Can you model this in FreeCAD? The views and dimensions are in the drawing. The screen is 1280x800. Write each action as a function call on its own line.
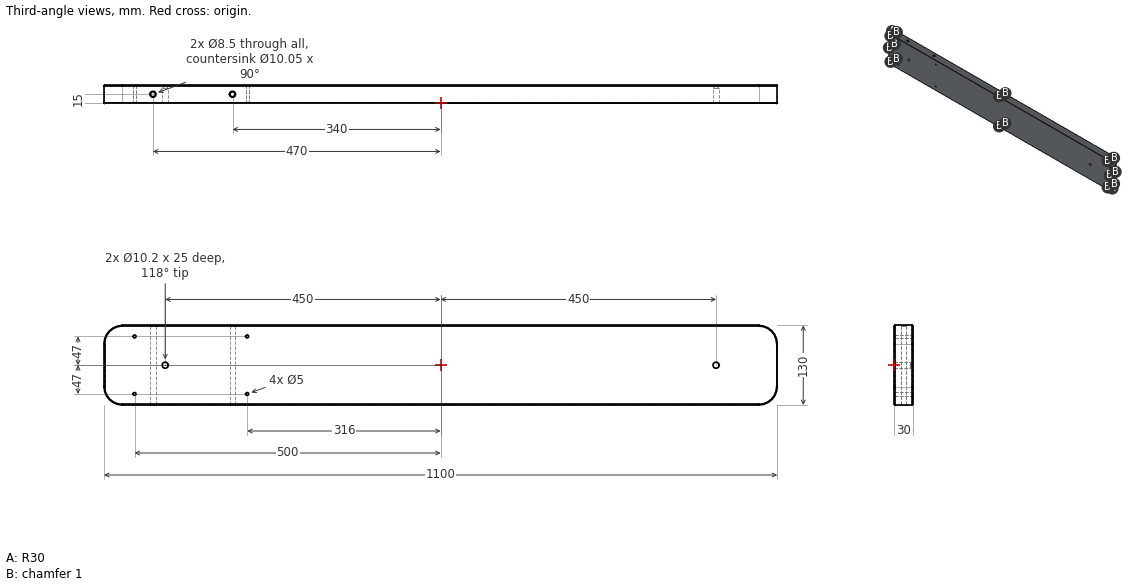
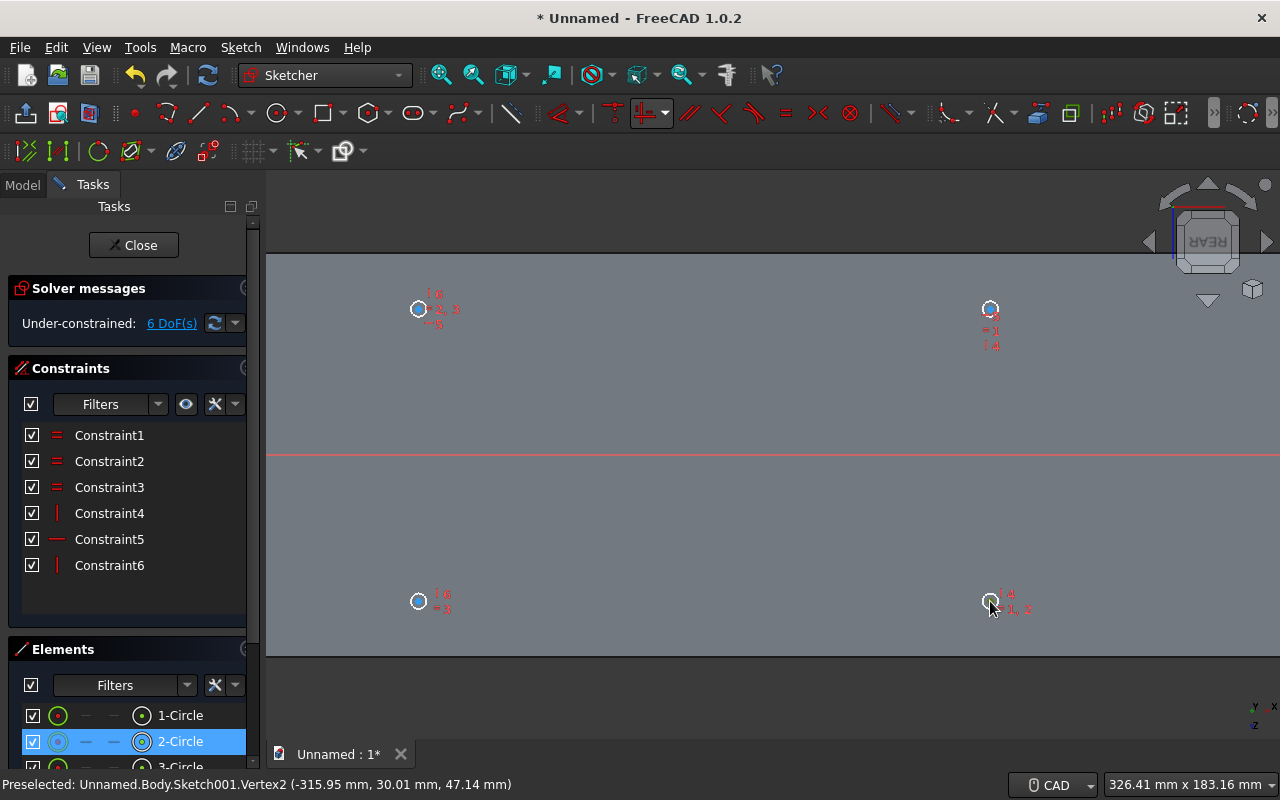
click(419, 601)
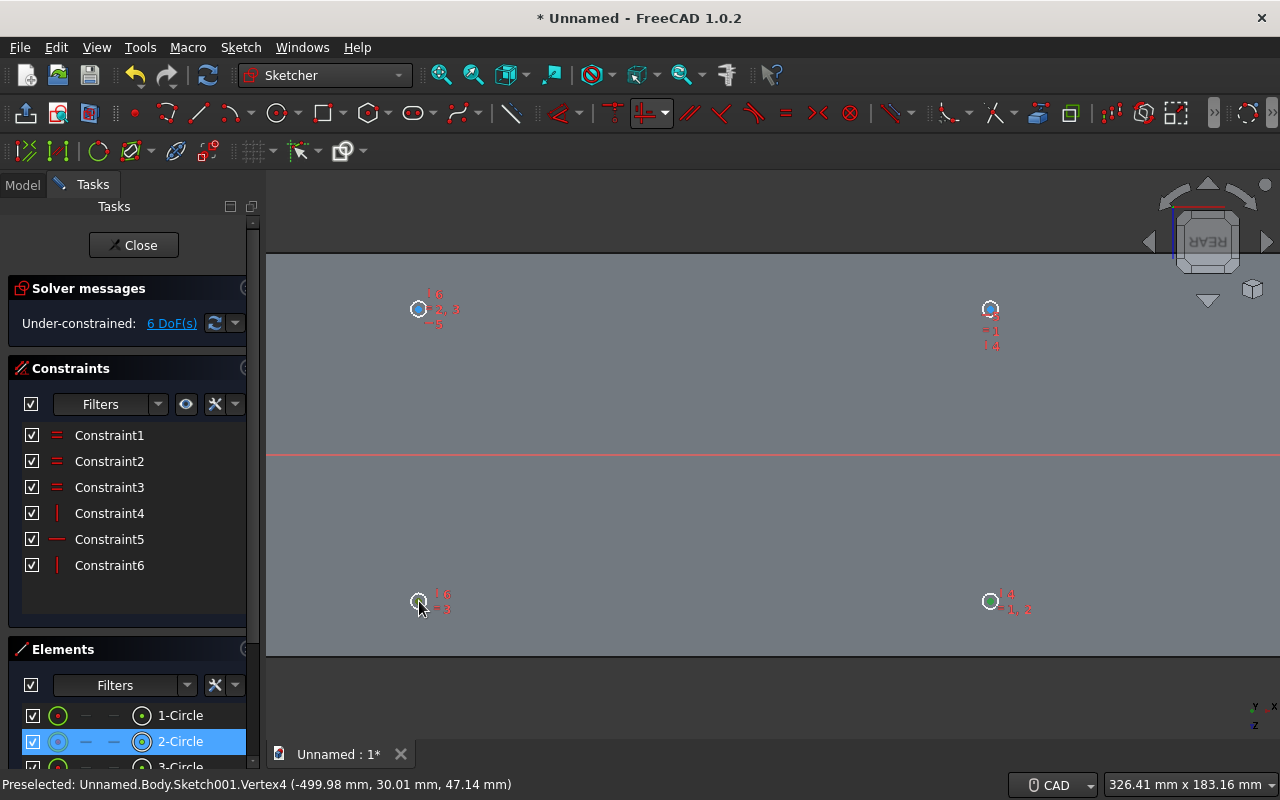
click(668, 114)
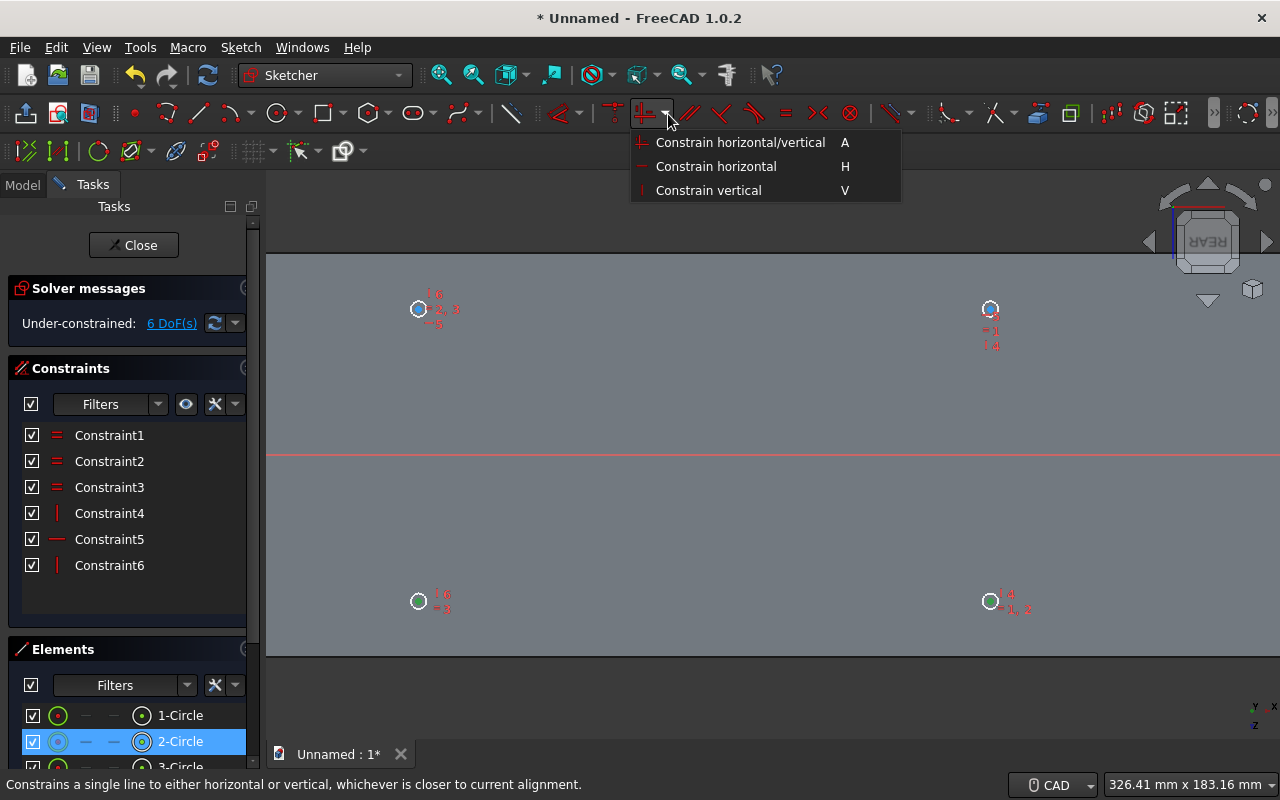
click(766, 166)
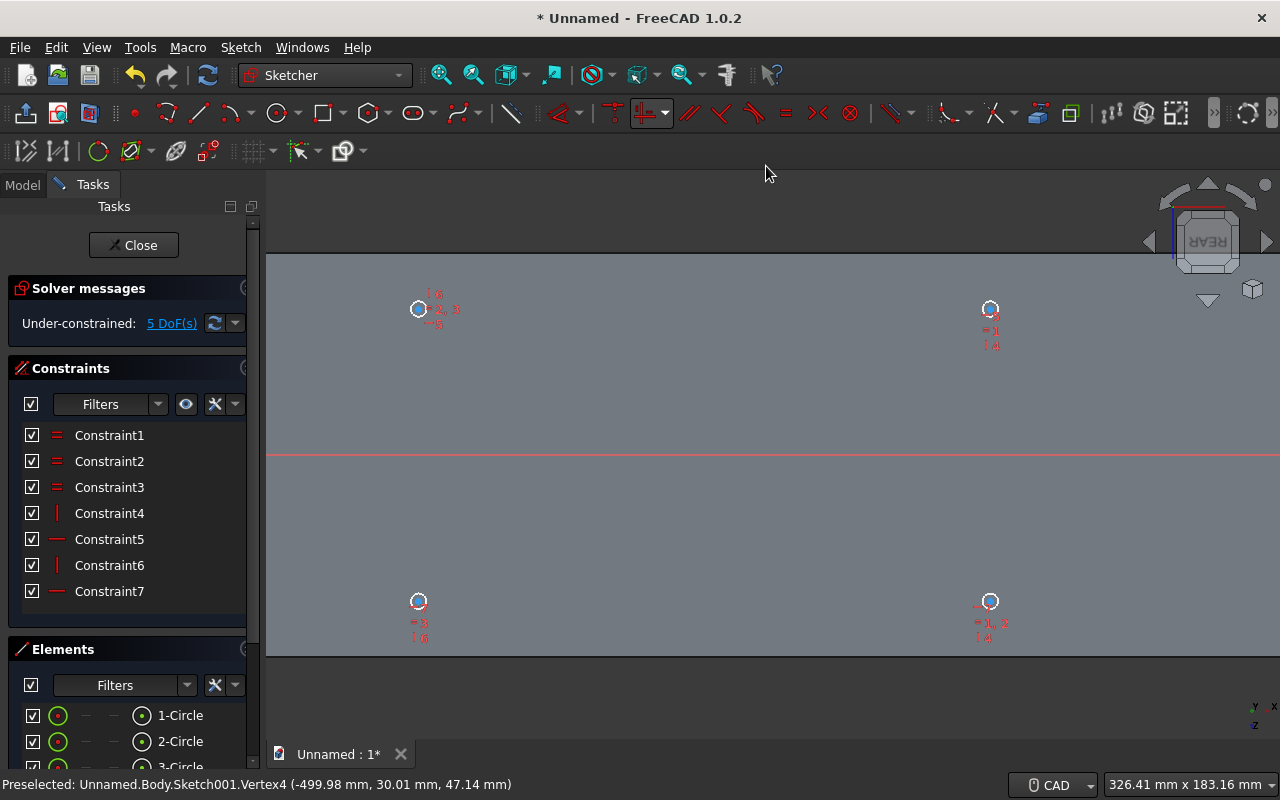
click(558, 114)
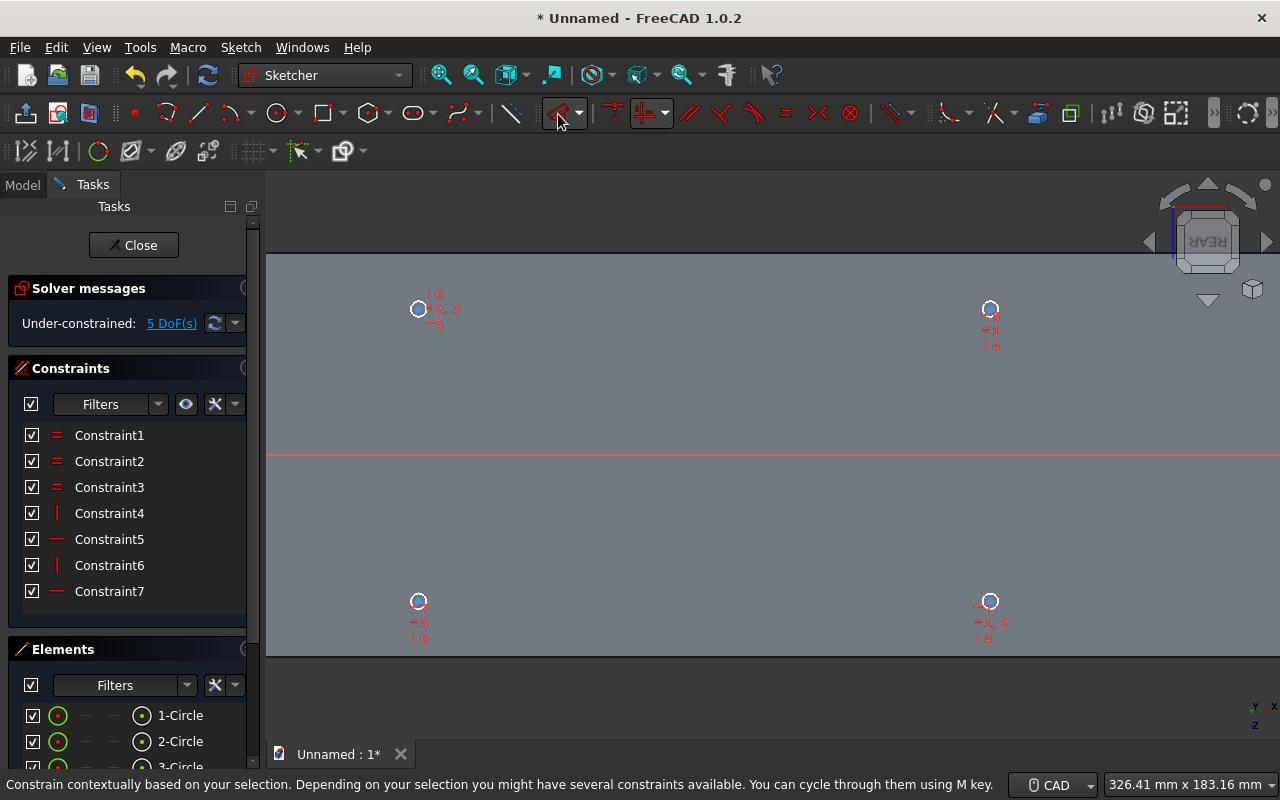
scroll(991, 301, up, 5)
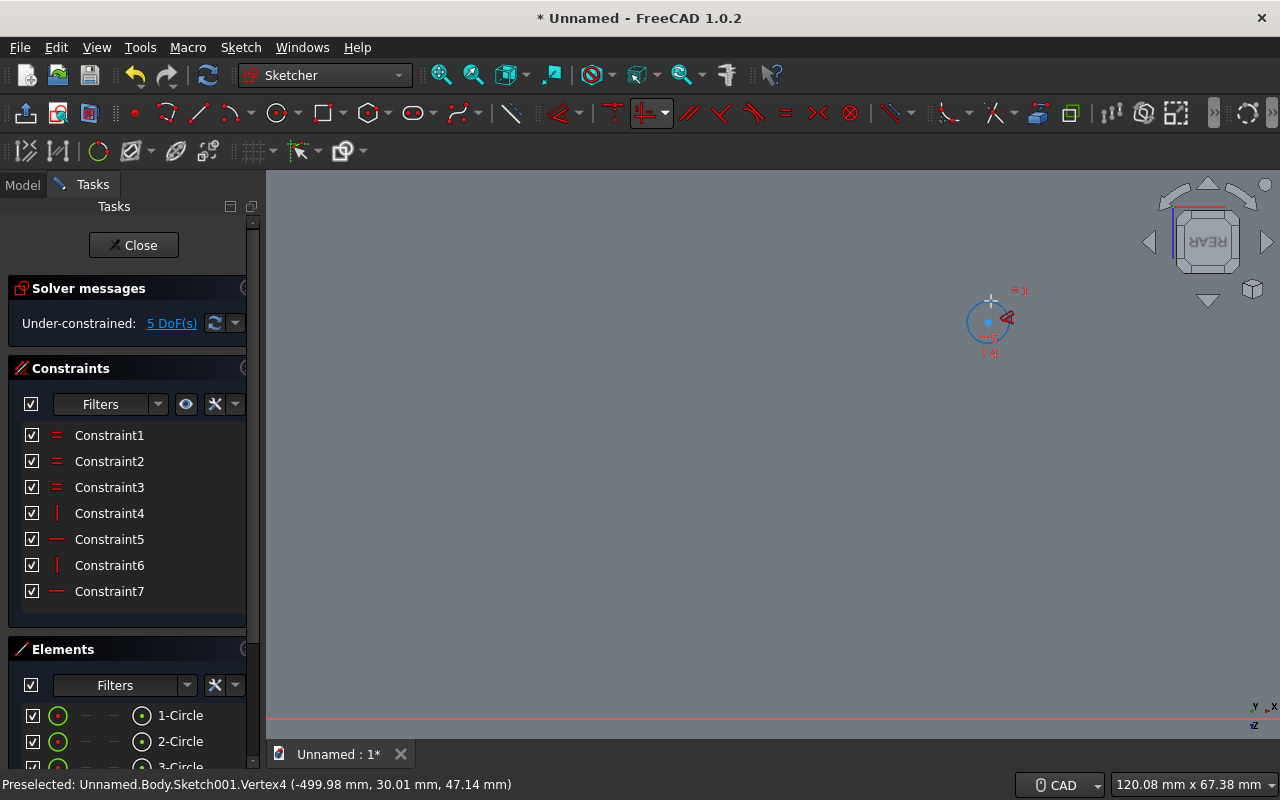
click(989, 302)
click(990, 270)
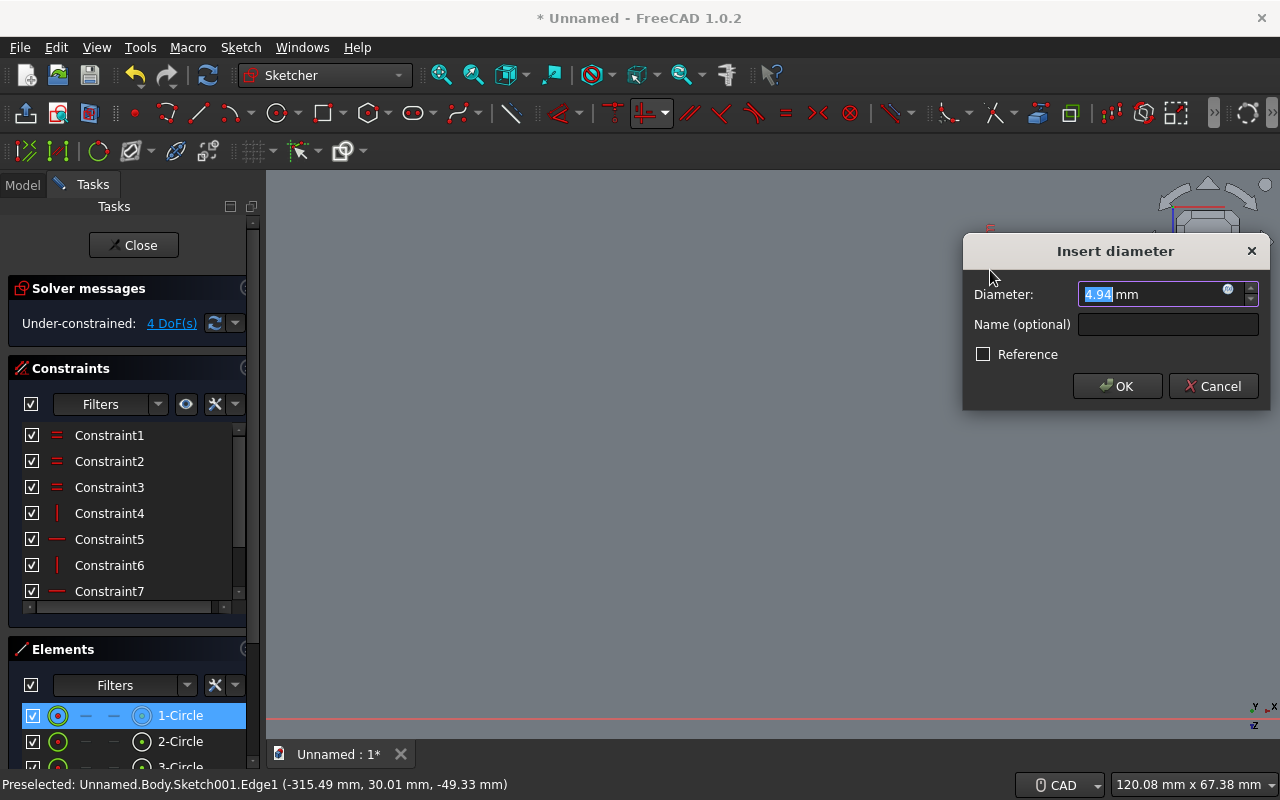
text(5)
key(Return)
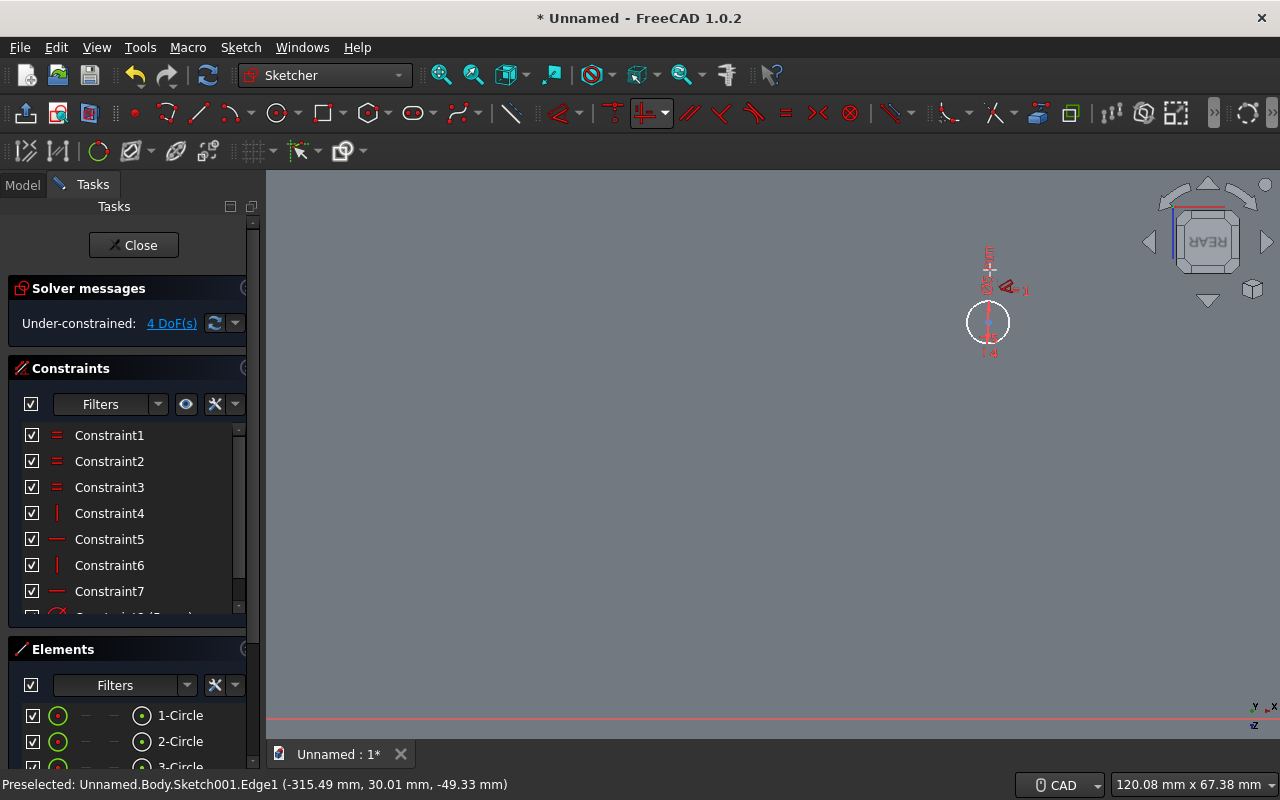
click(988, 322)
click(954, 517)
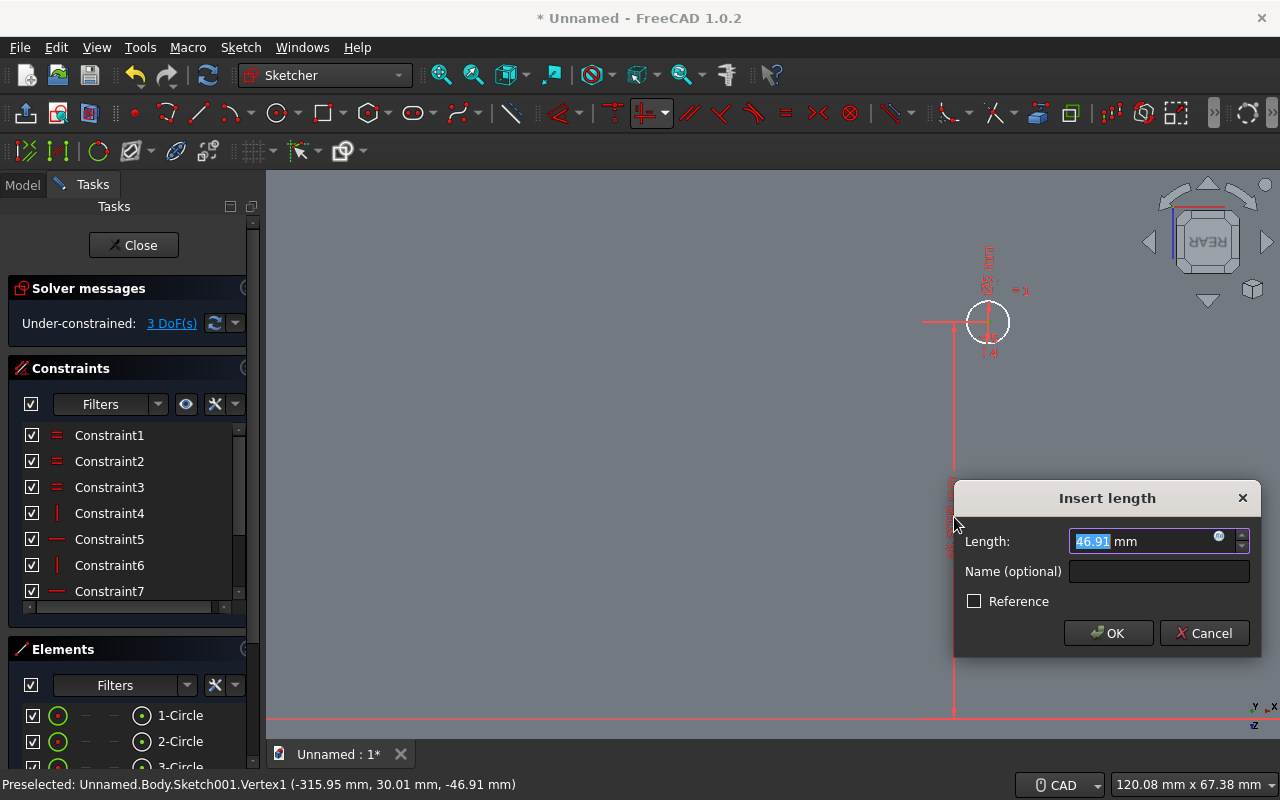
text(47)
key(Return)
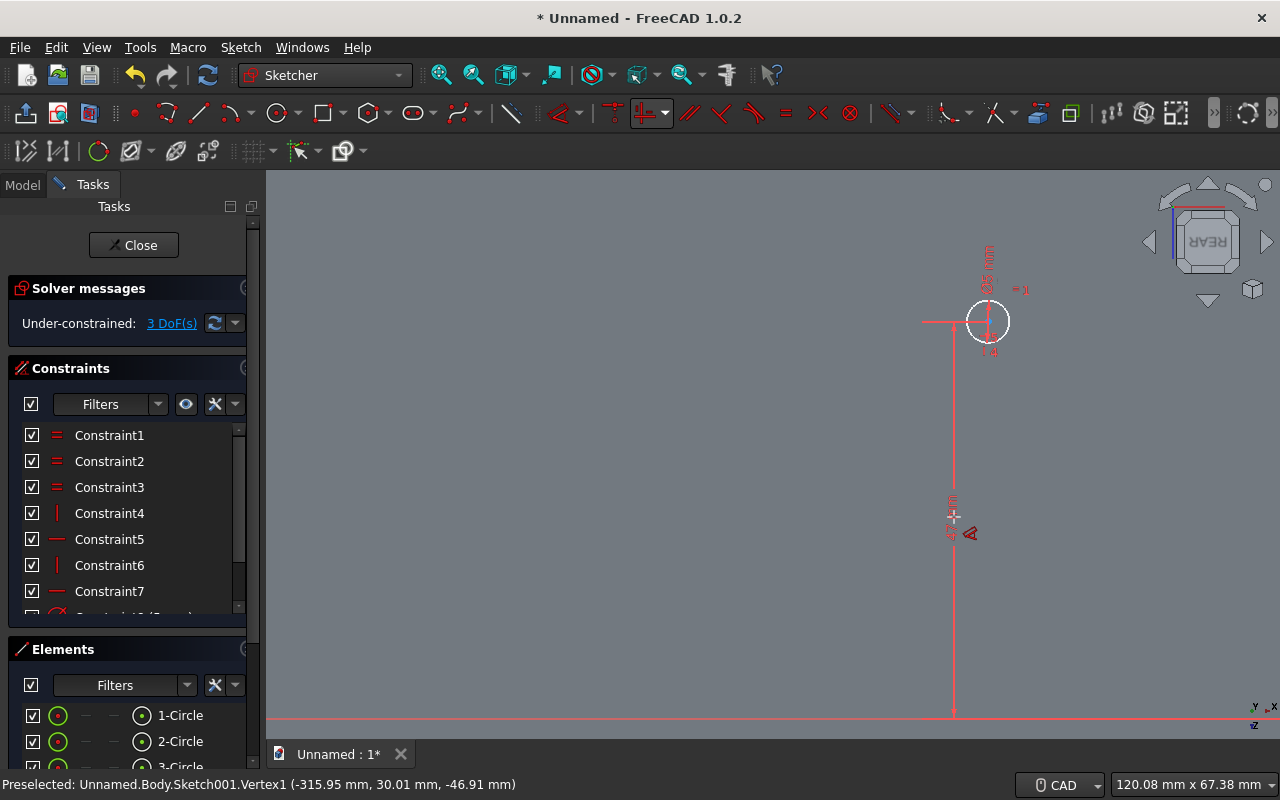
scroll(992, 301, down, 5)